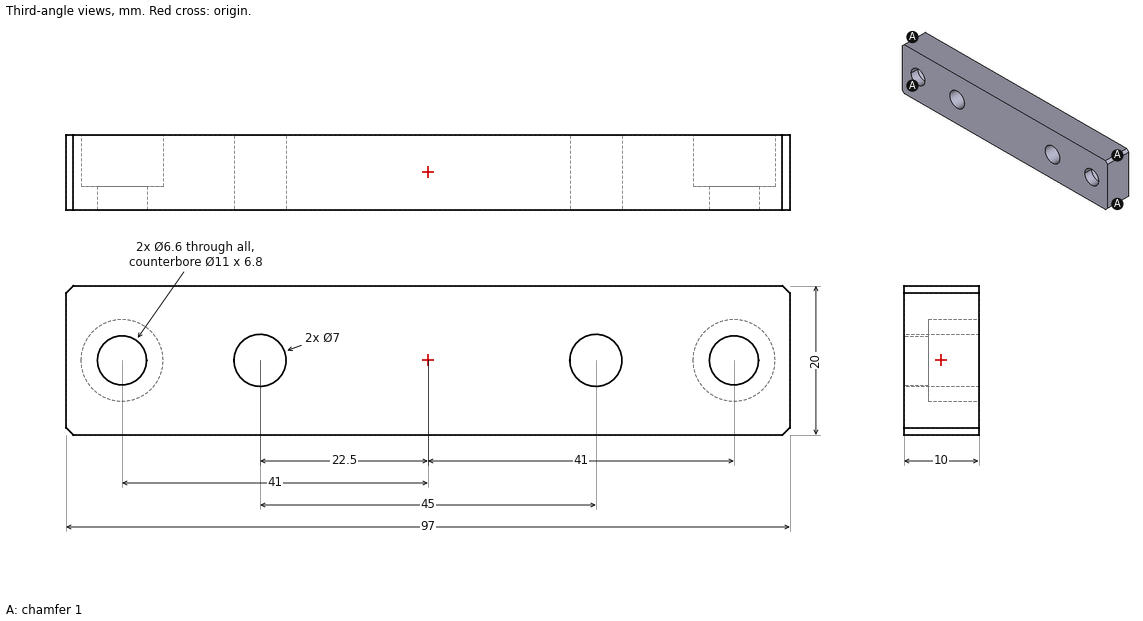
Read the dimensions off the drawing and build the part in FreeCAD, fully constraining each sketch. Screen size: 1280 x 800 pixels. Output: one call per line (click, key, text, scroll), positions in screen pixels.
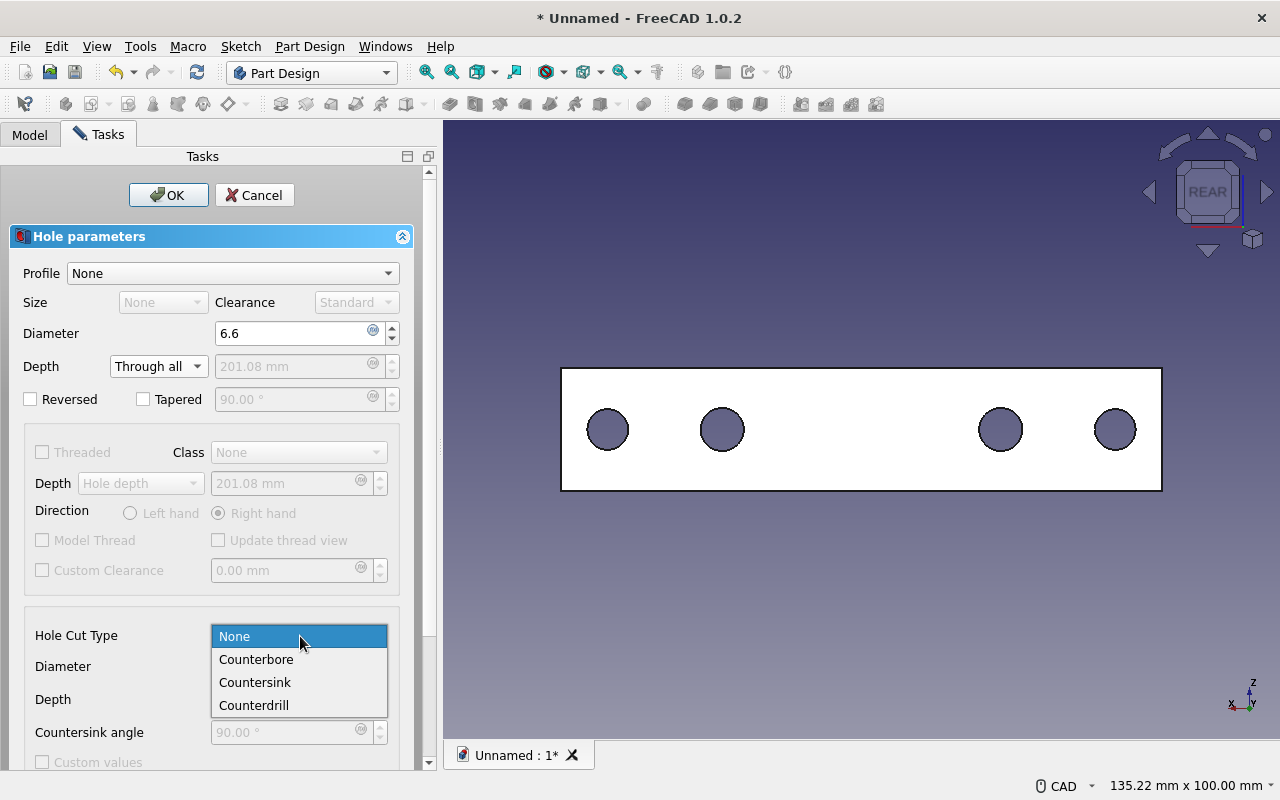
click(298, 660)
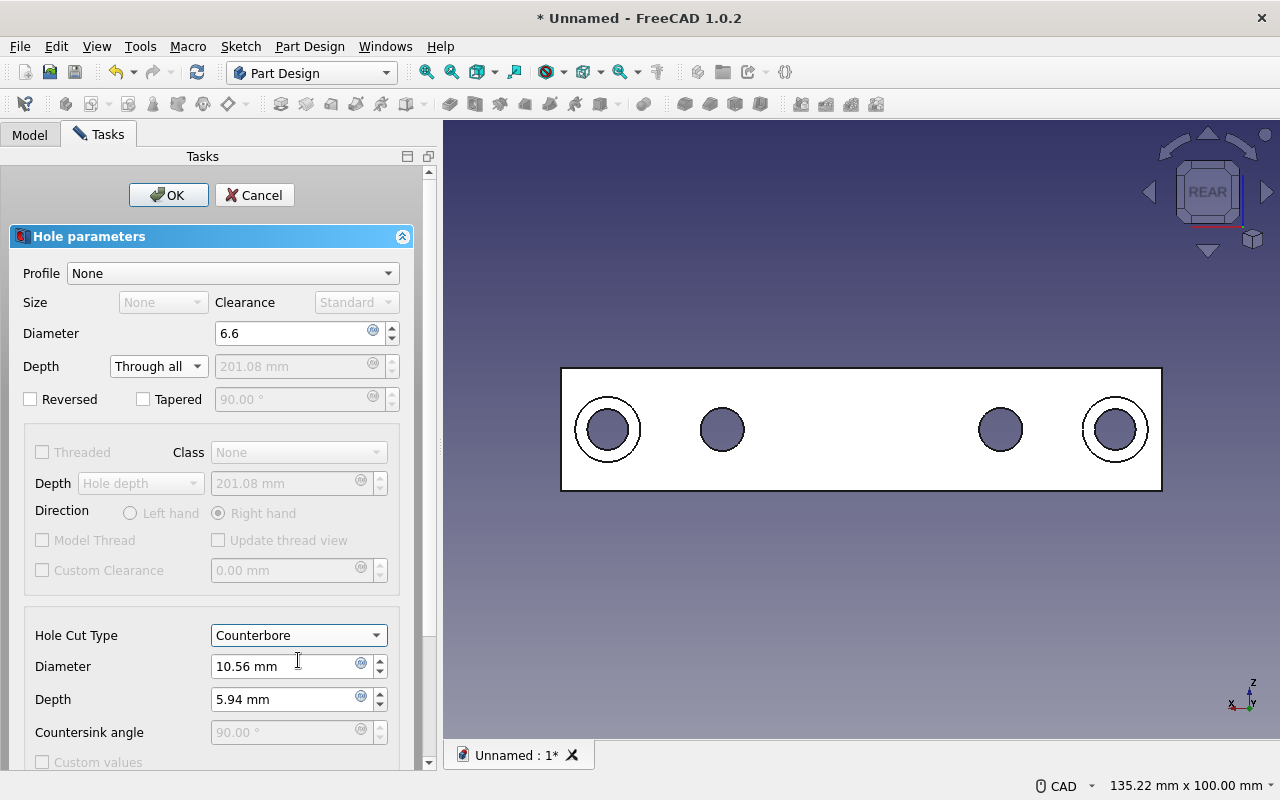
triple_click(292, 666)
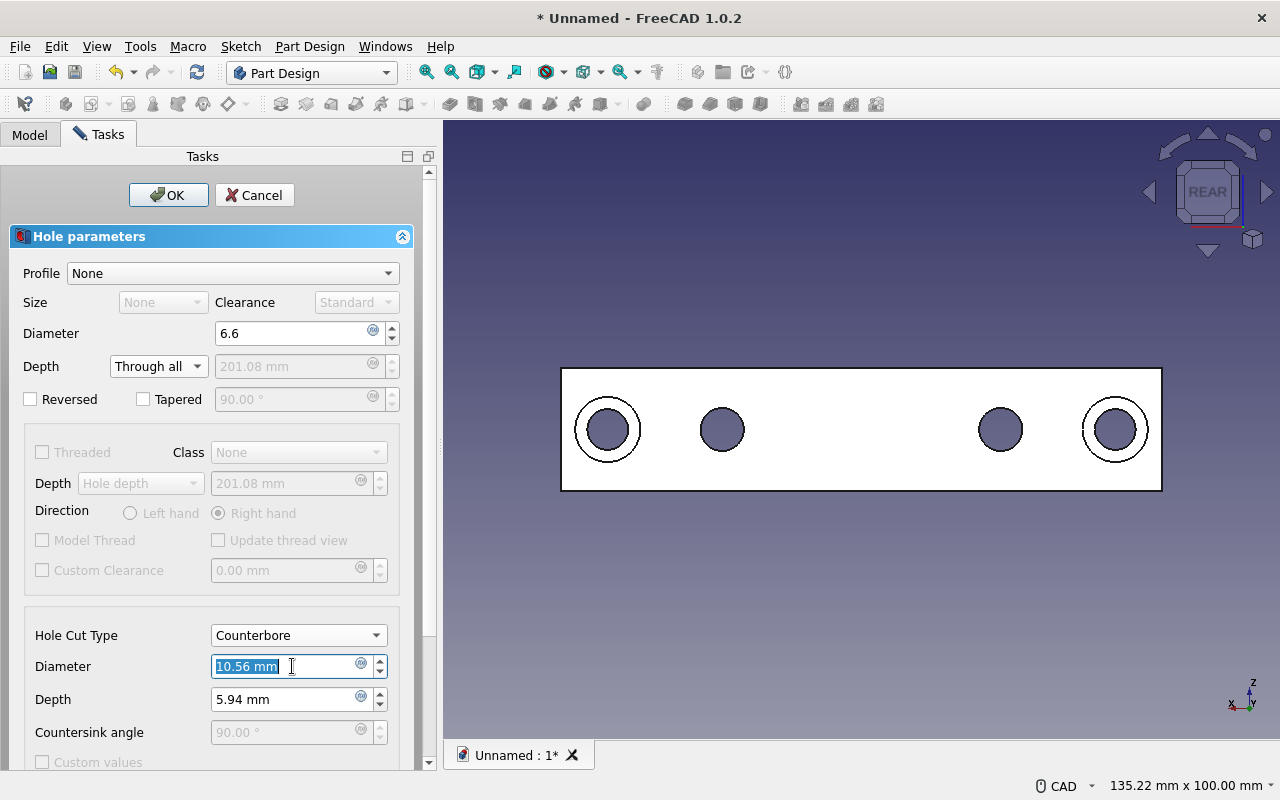
text(11)
key(Tab)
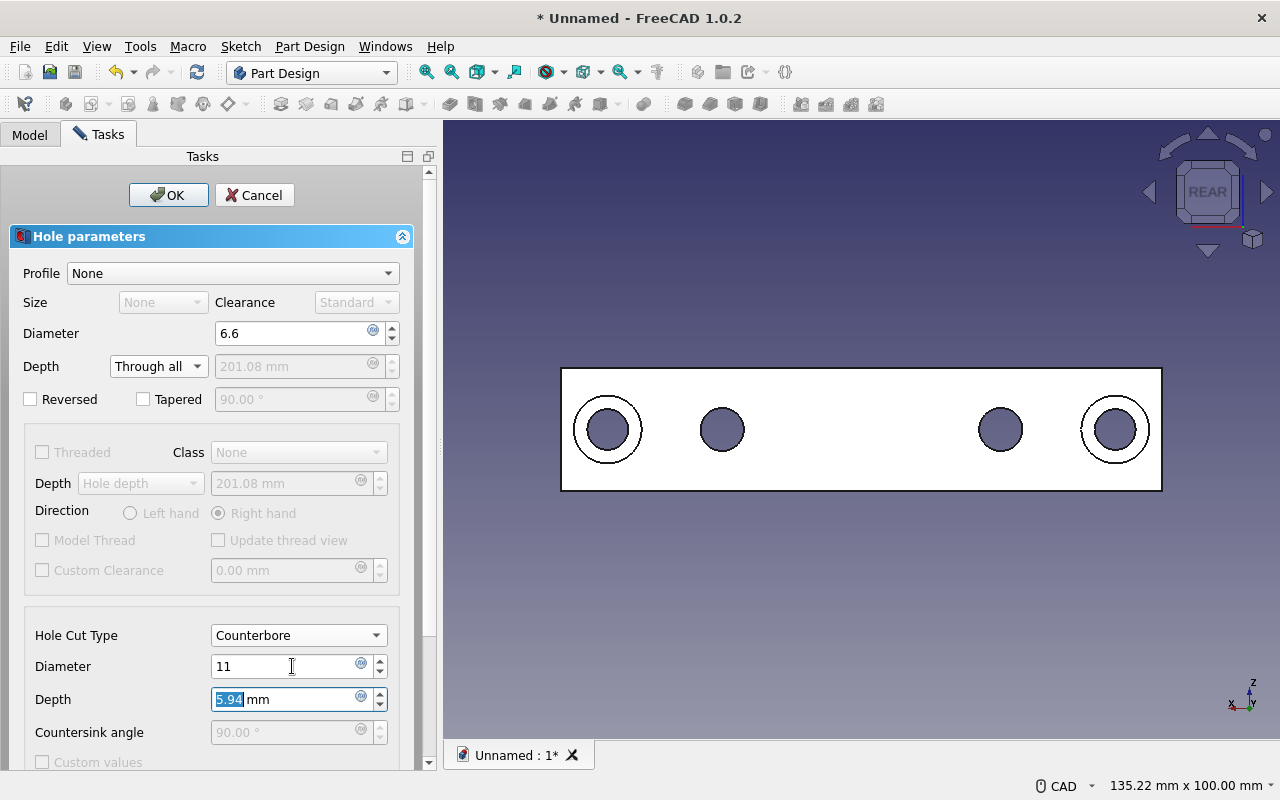
text(6.8)
key(Tab)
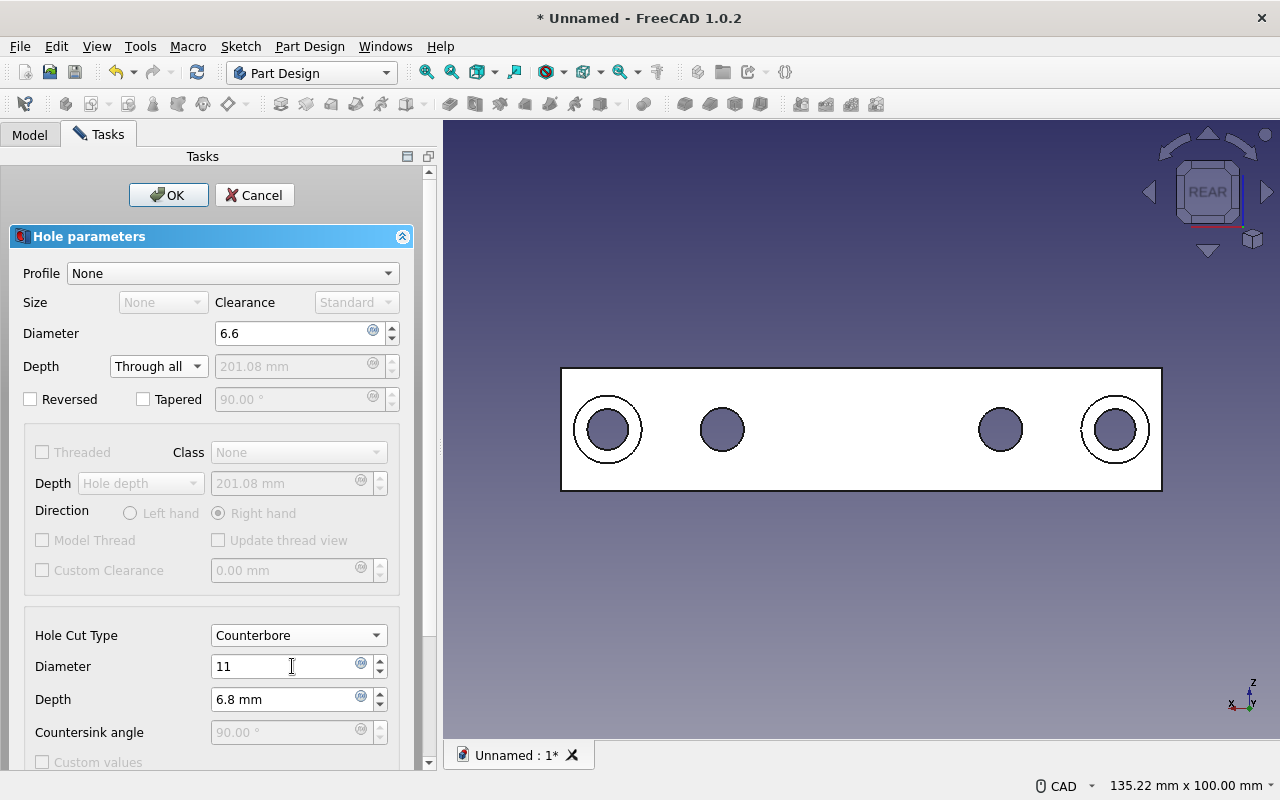
click(169, 195)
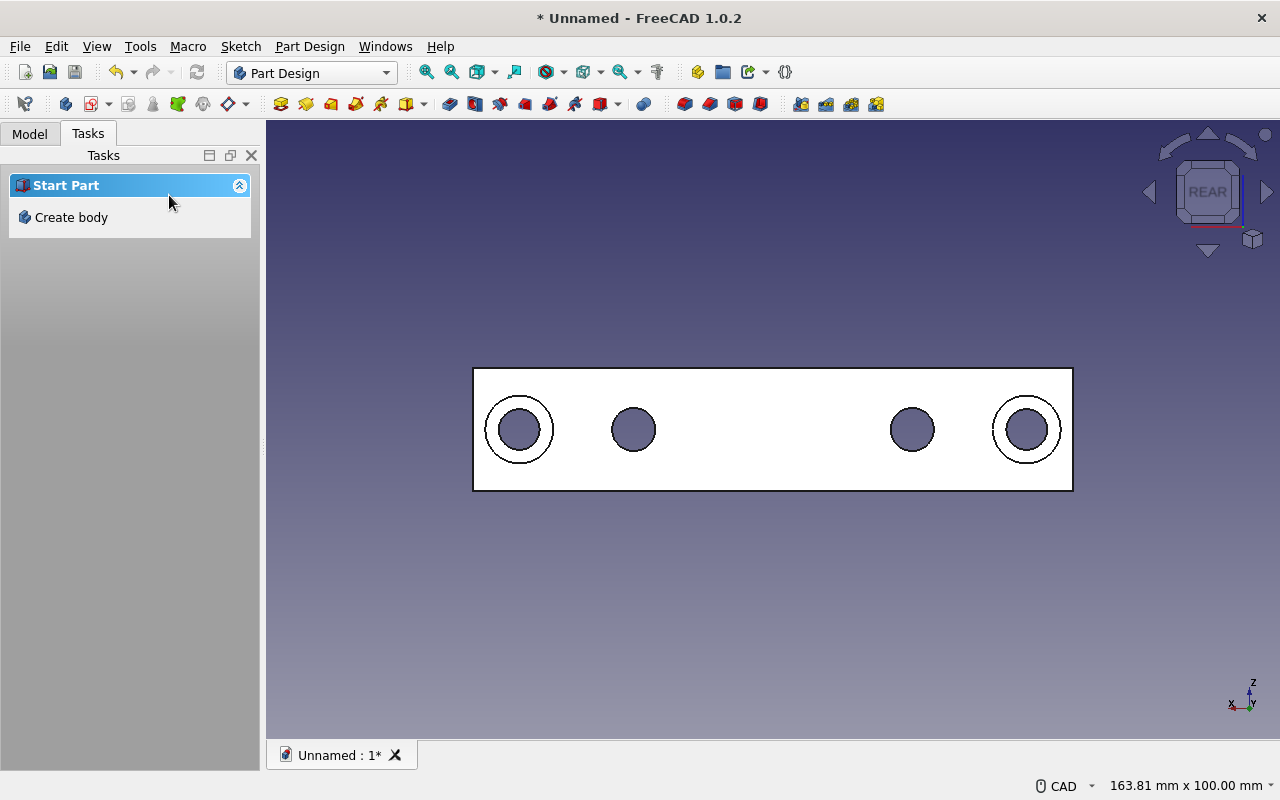
key(0)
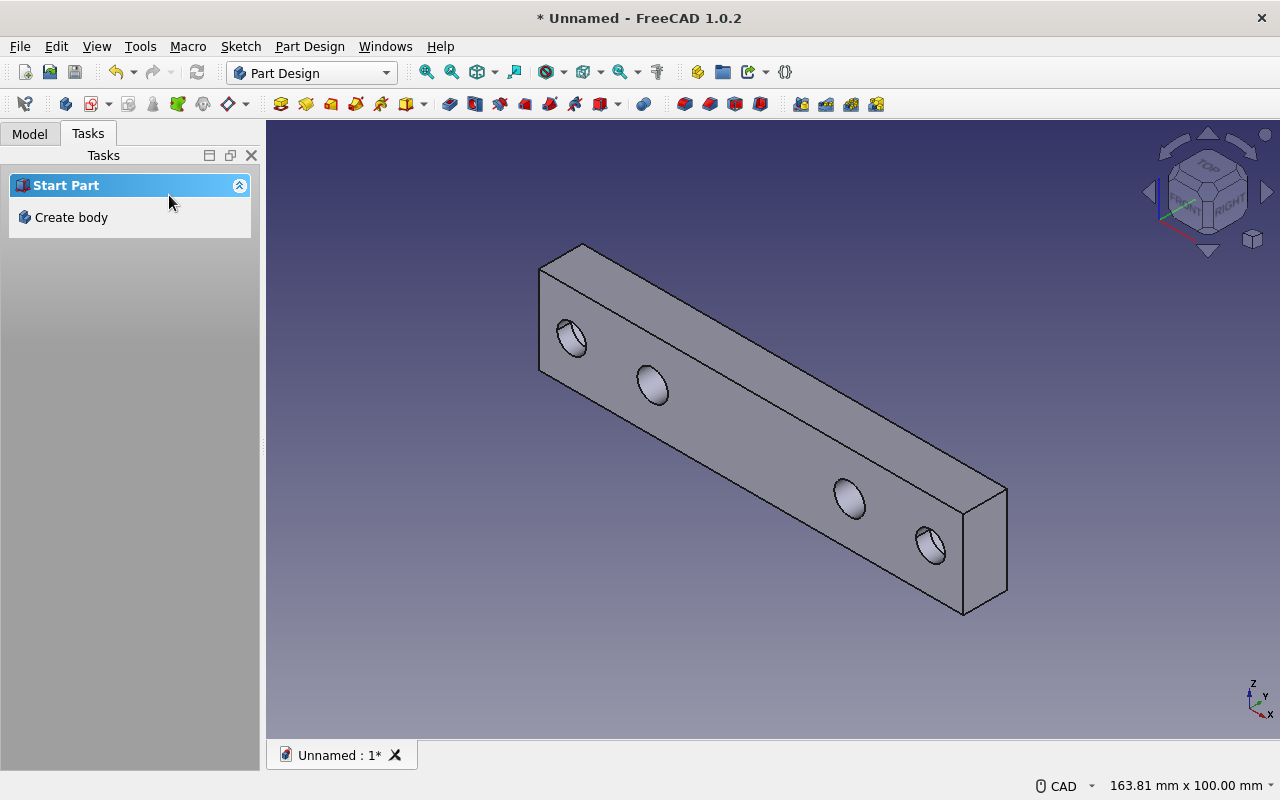
click(985, 501)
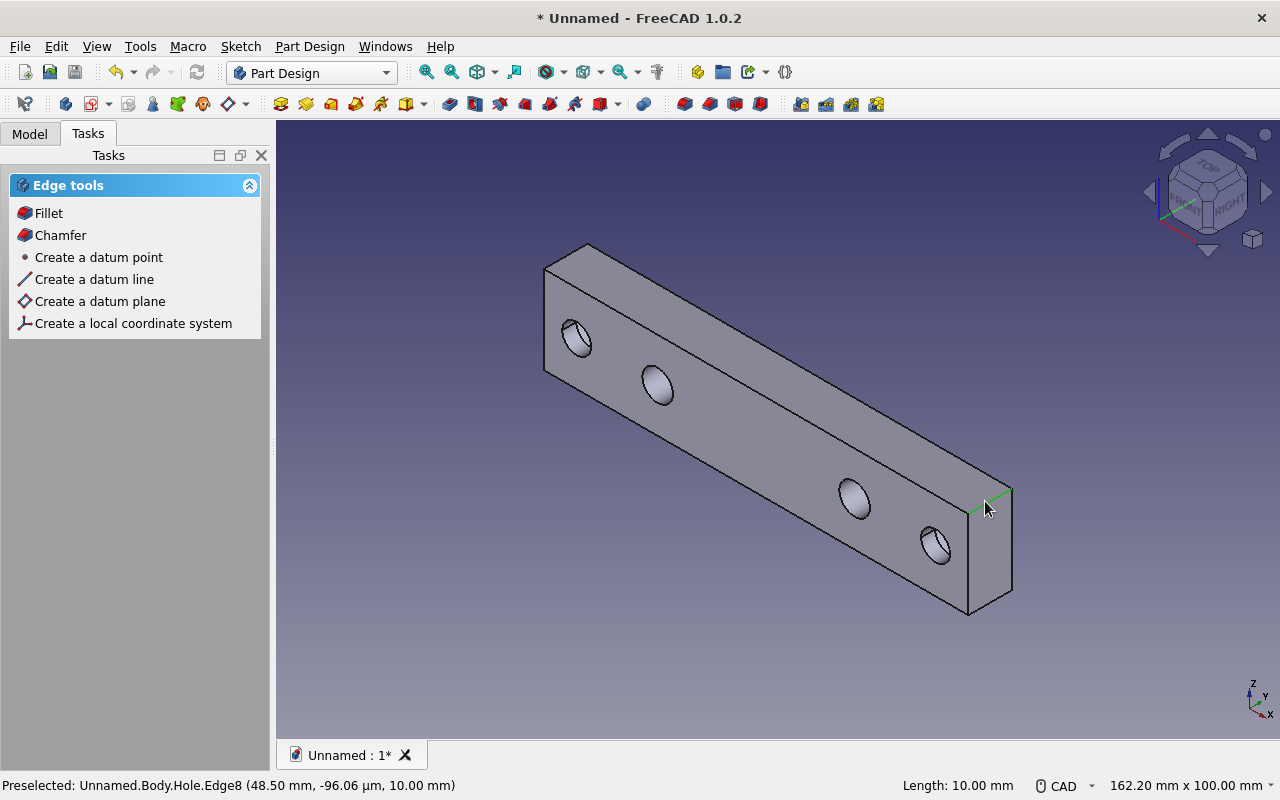
key(2)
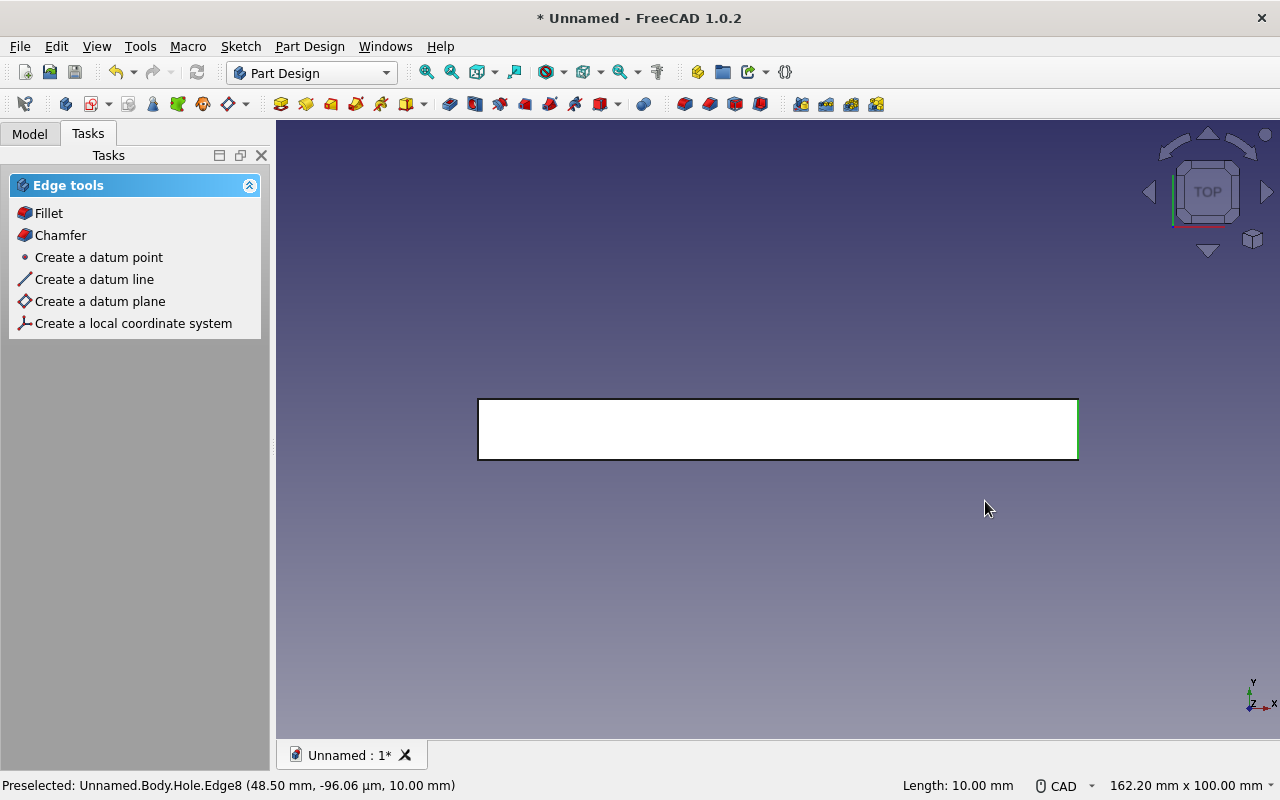
click(478, 428, ctrl)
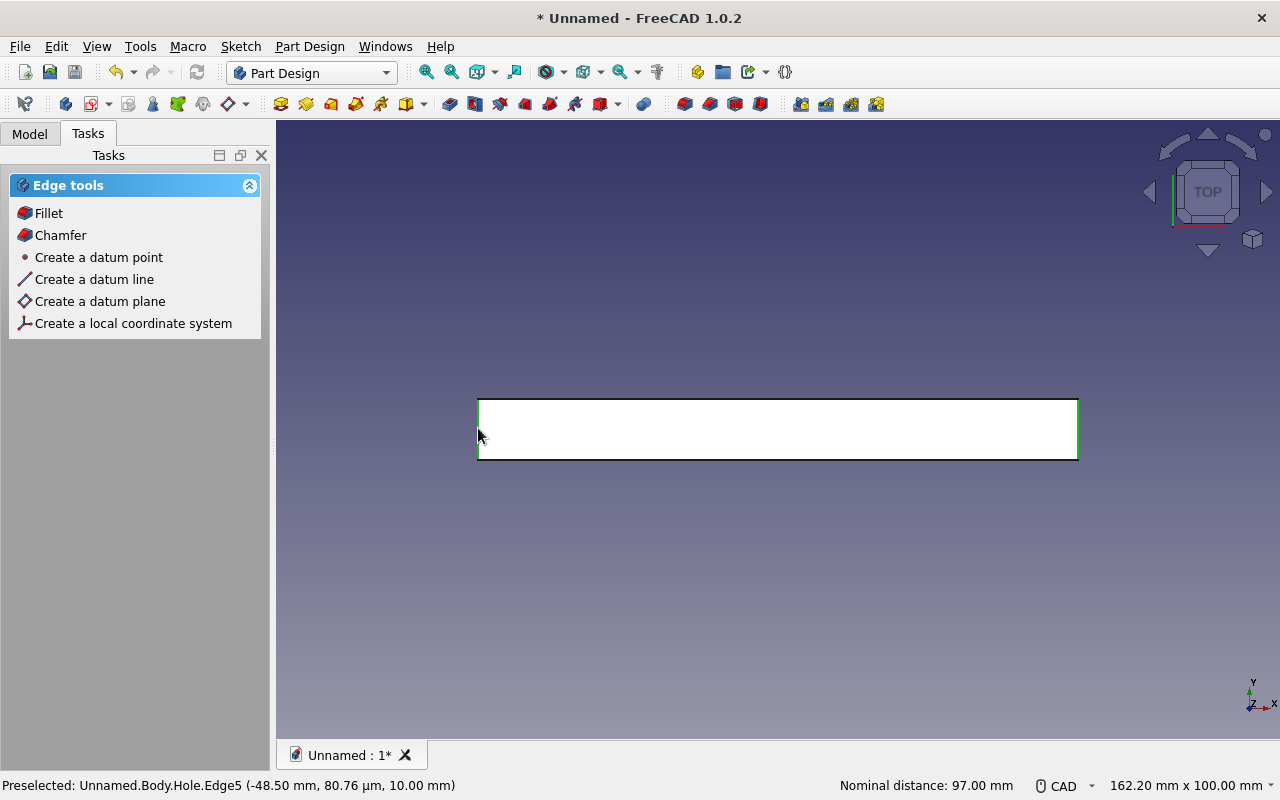
key(1)